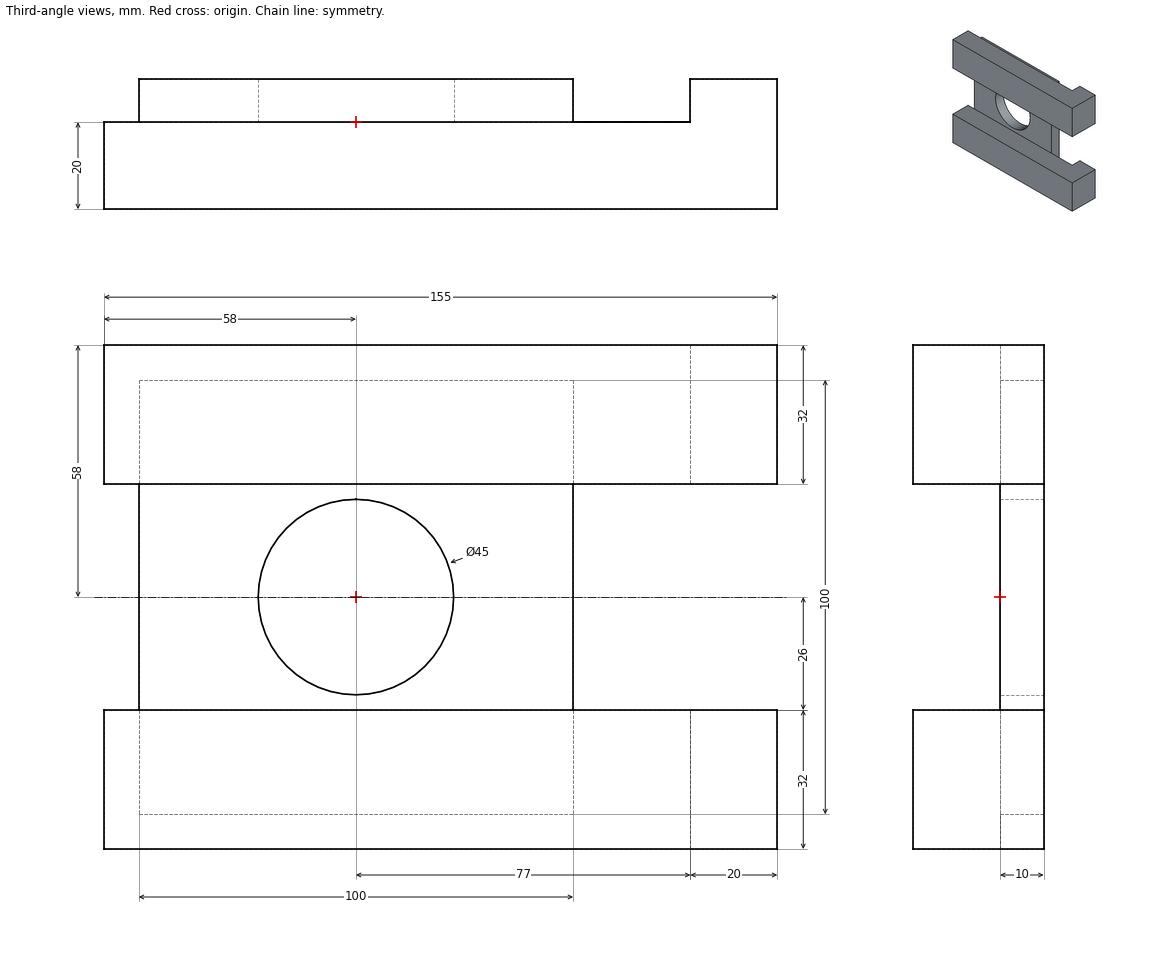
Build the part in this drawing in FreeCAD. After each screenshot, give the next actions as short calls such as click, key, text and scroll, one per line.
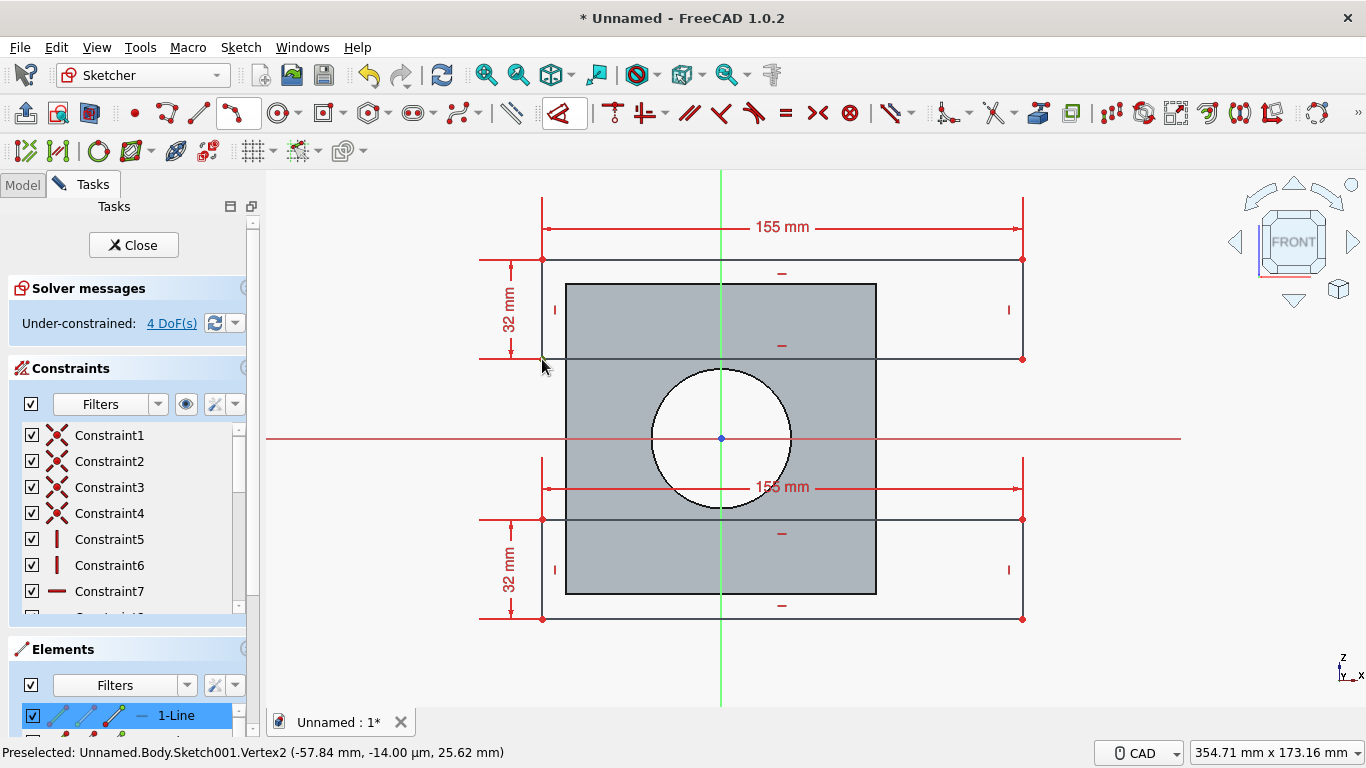
click(542, 520)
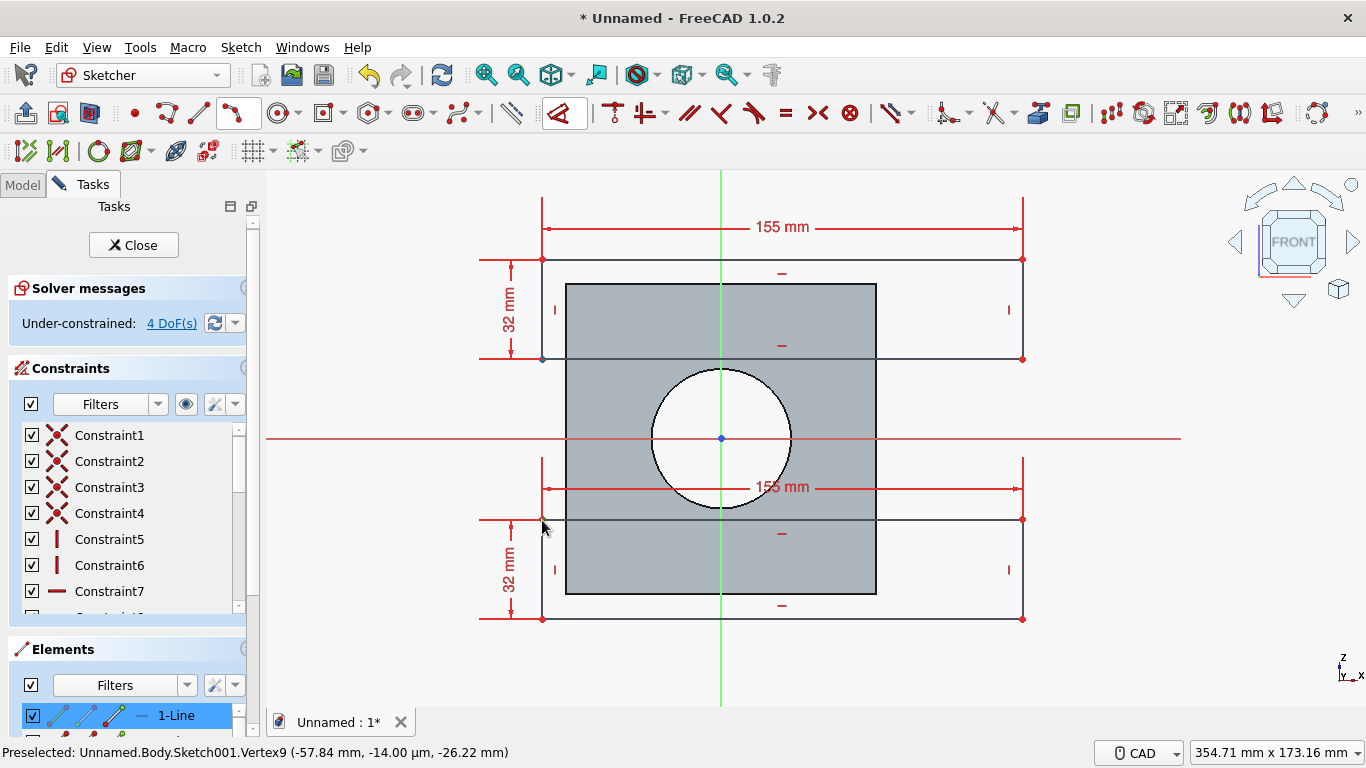
click(359, 439)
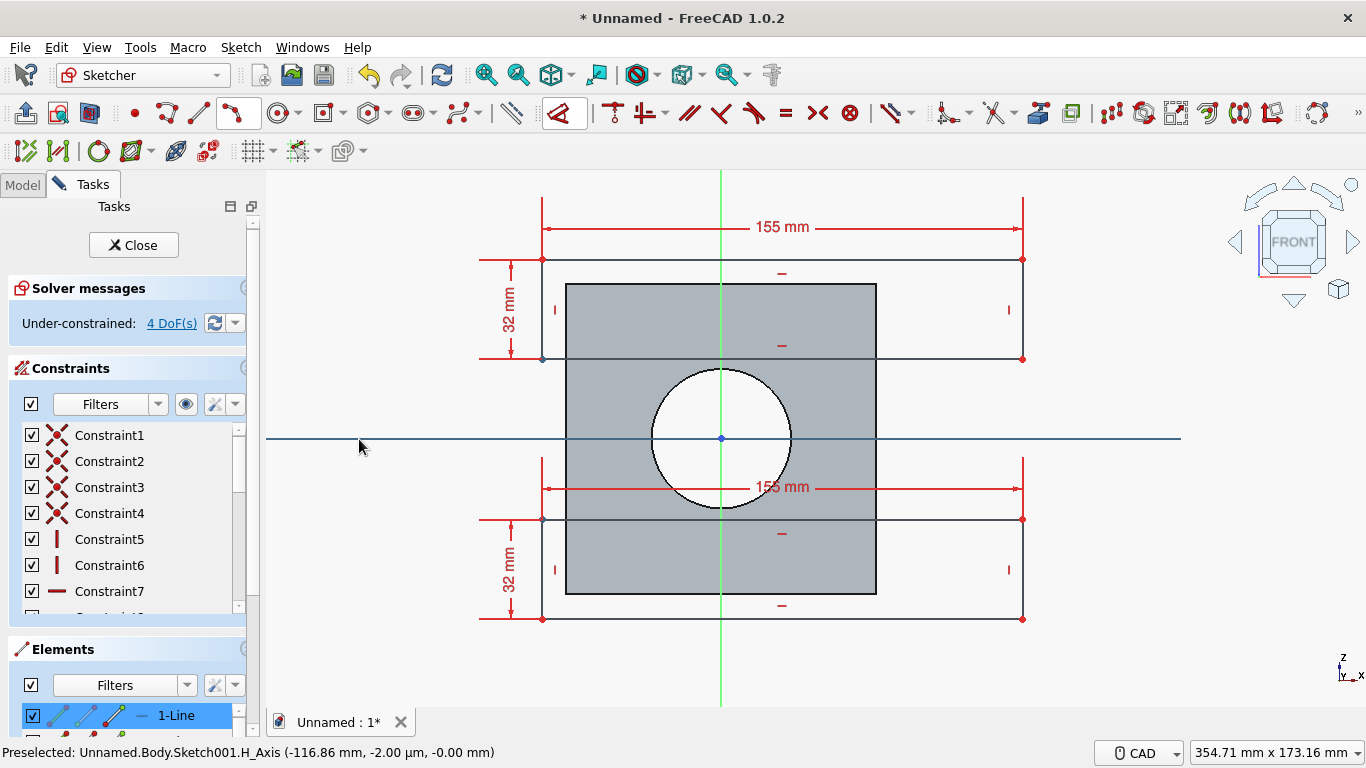
key(s)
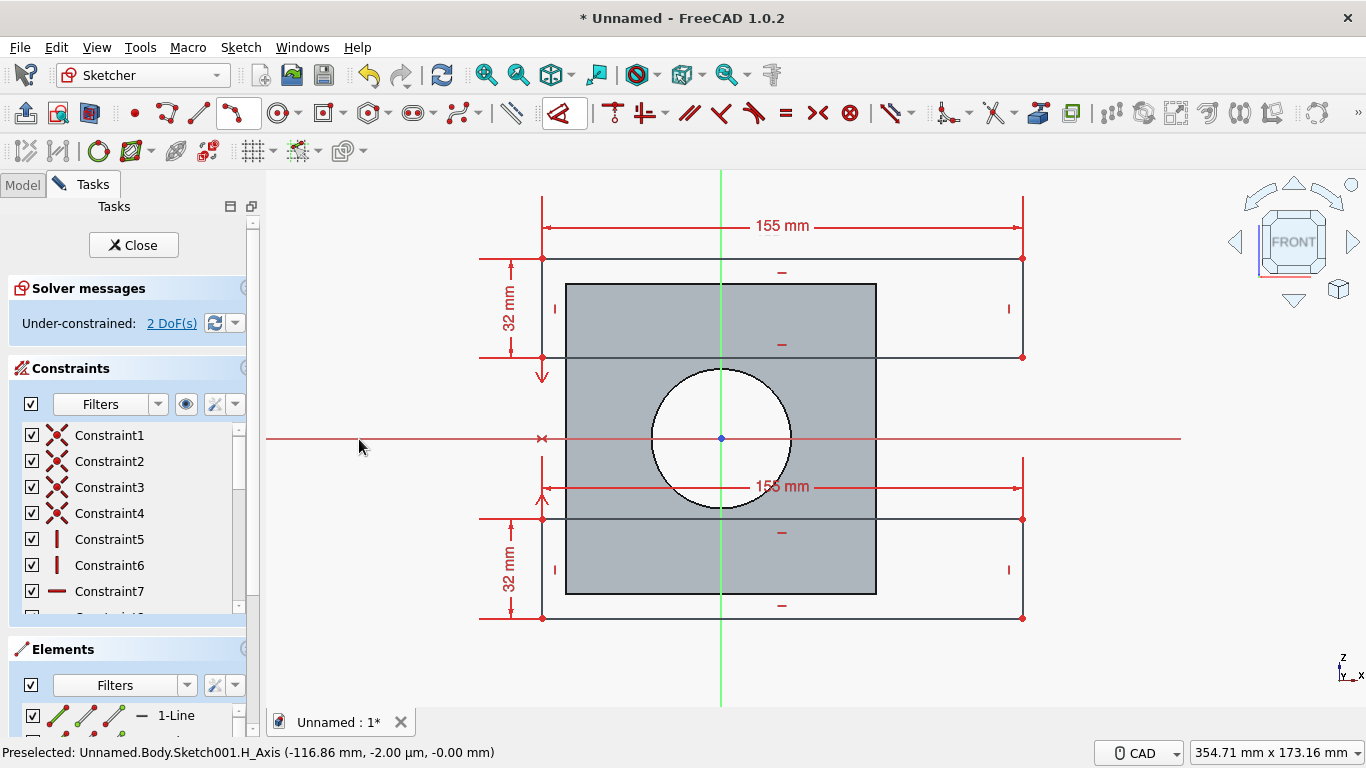
key(d)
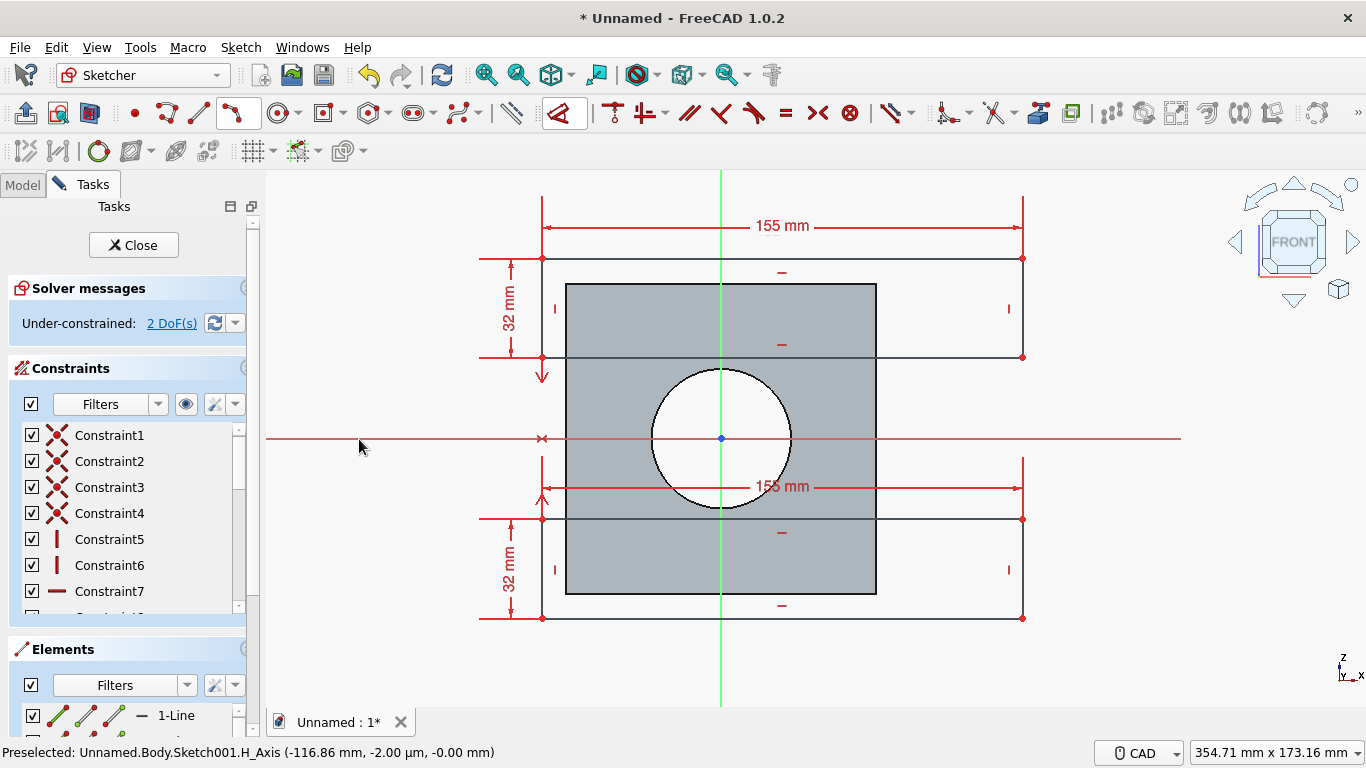
click(542, 259)
click(632, 225)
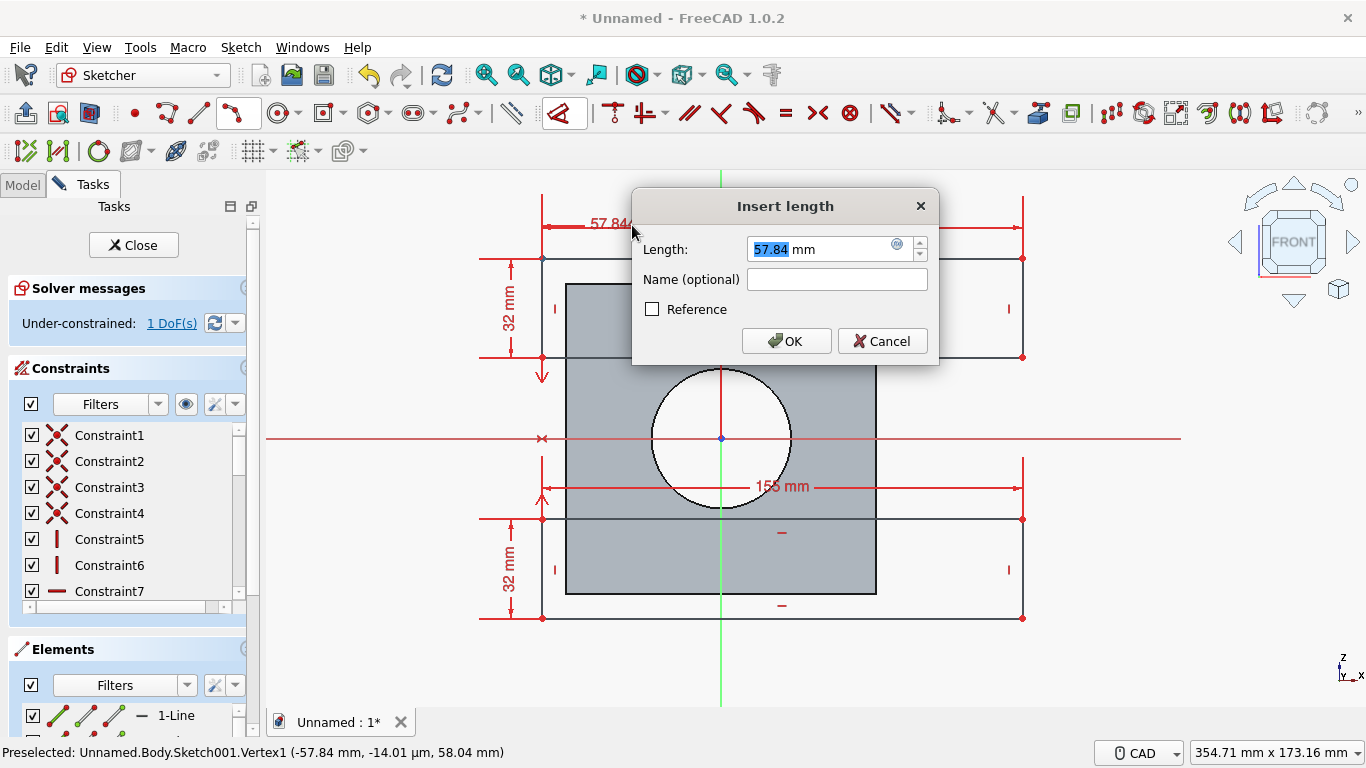
text(58)
key(Return)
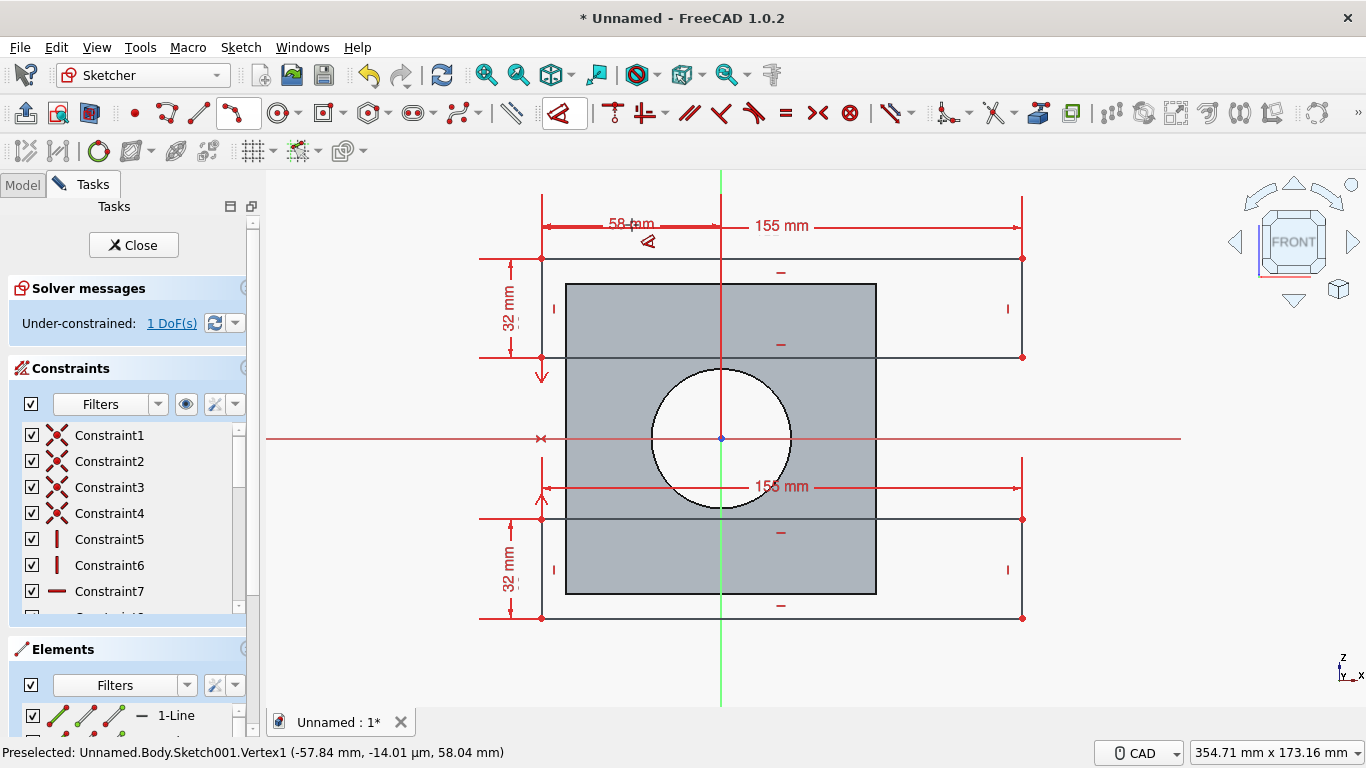
click(542, 259)
click(508, 349)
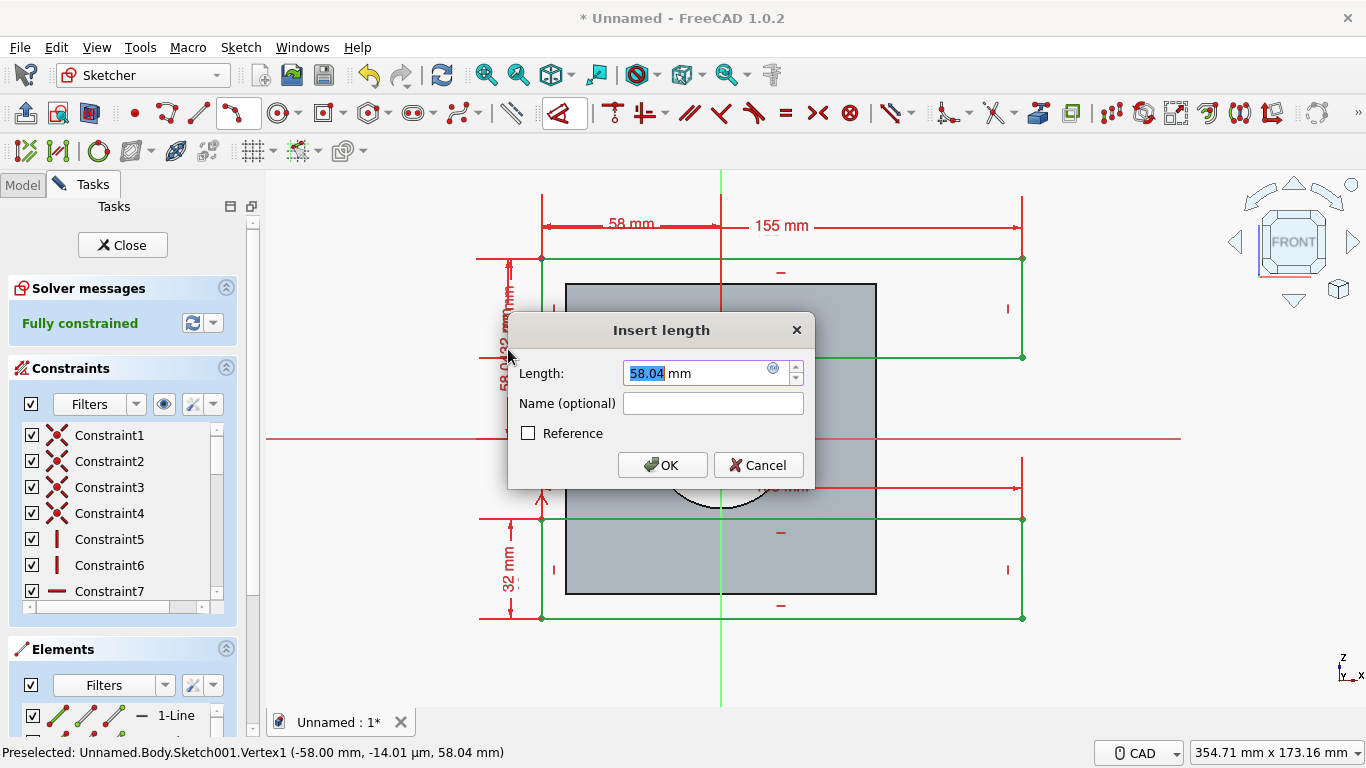
text(58)
key(Return)
key(Escape)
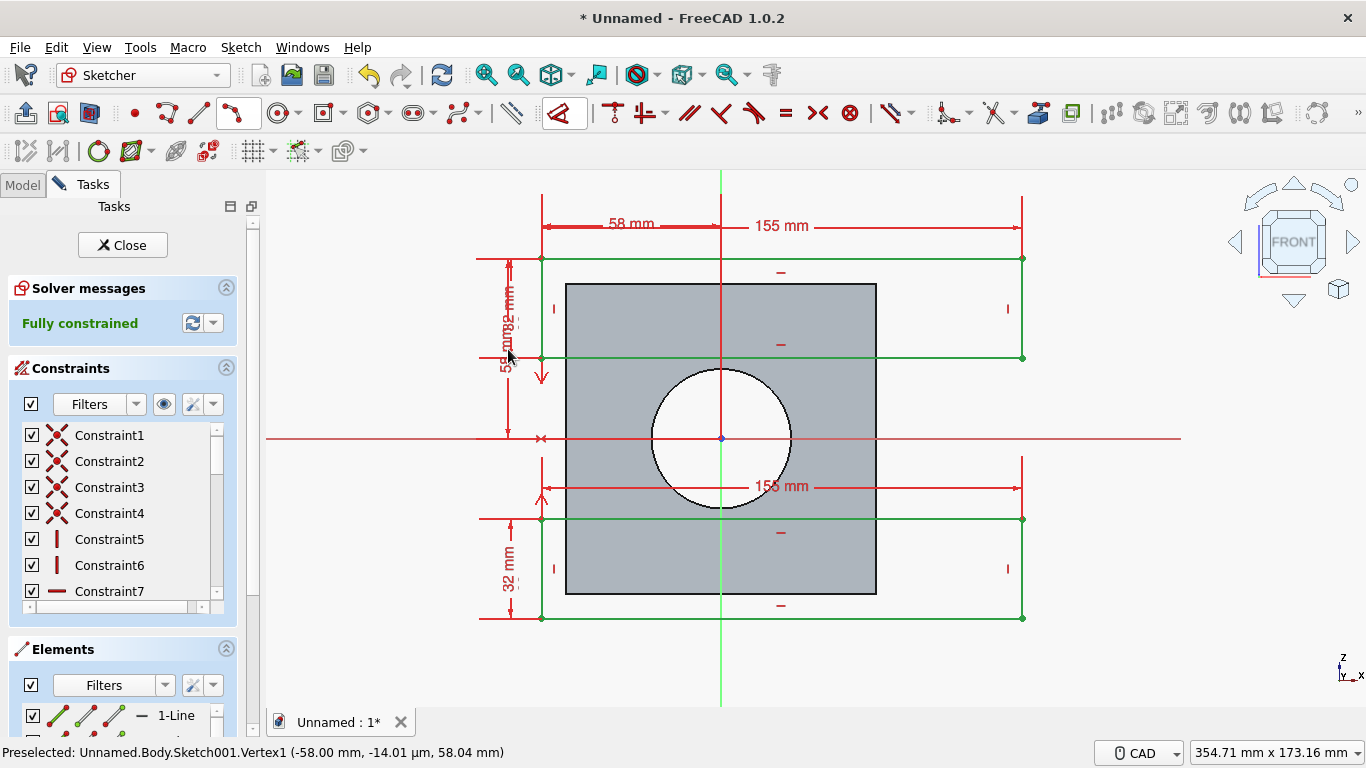
click(123, 245)